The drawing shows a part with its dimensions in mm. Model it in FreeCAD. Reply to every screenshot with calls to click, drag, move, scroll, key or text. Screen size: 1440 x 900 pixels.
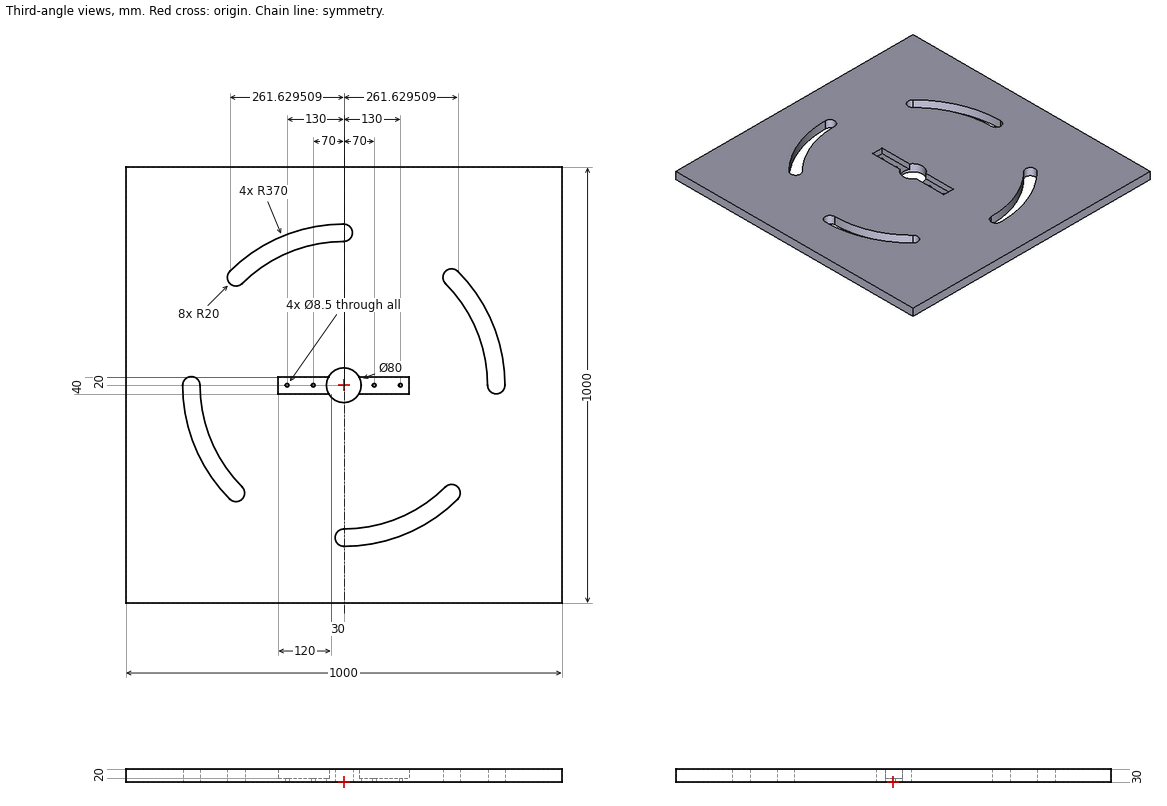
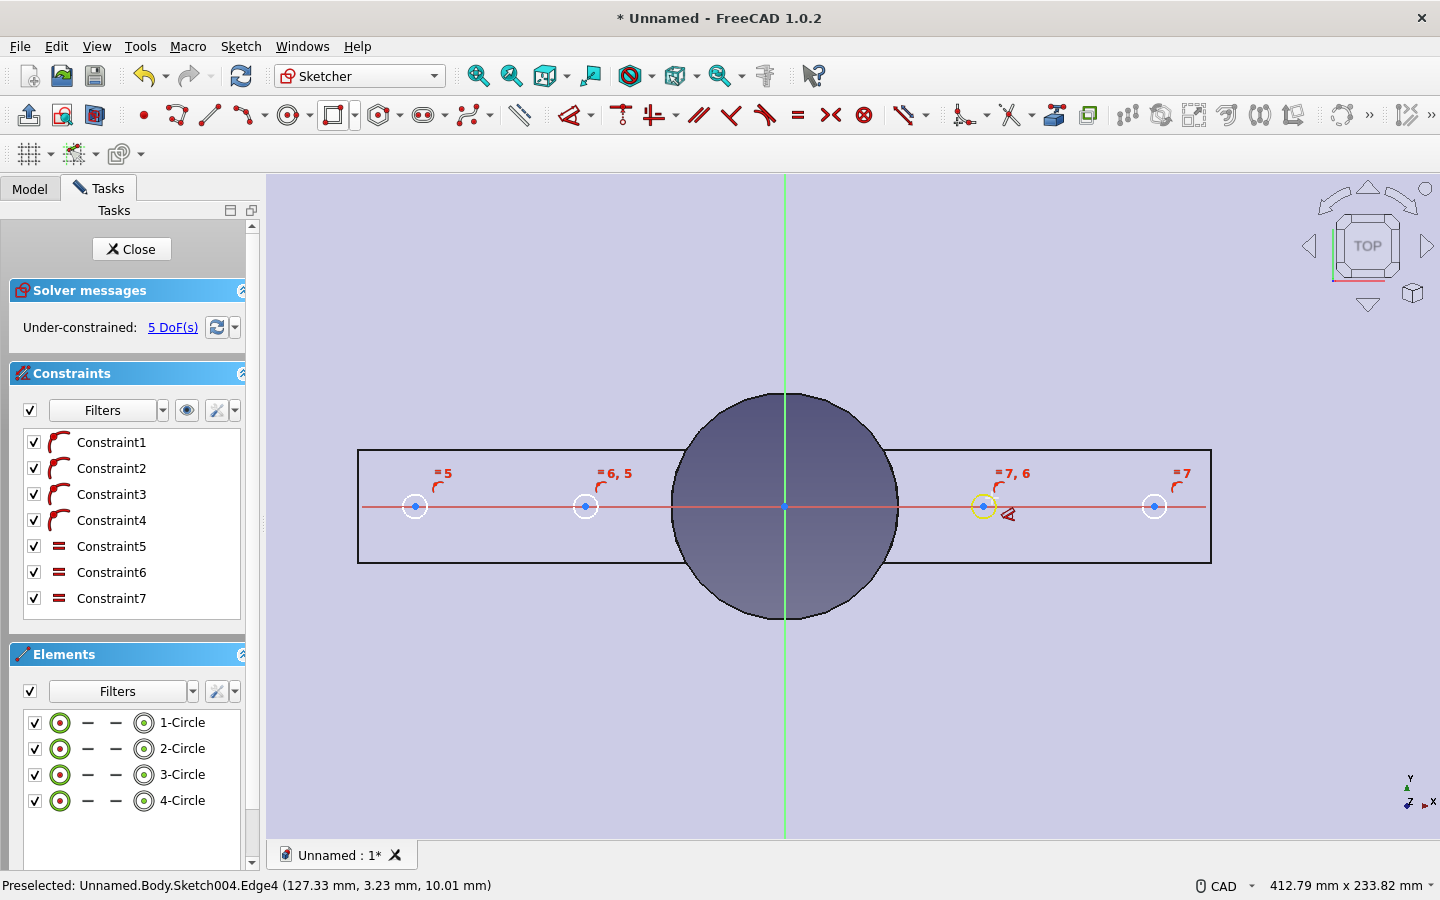
scroll(423, 498, up, 3)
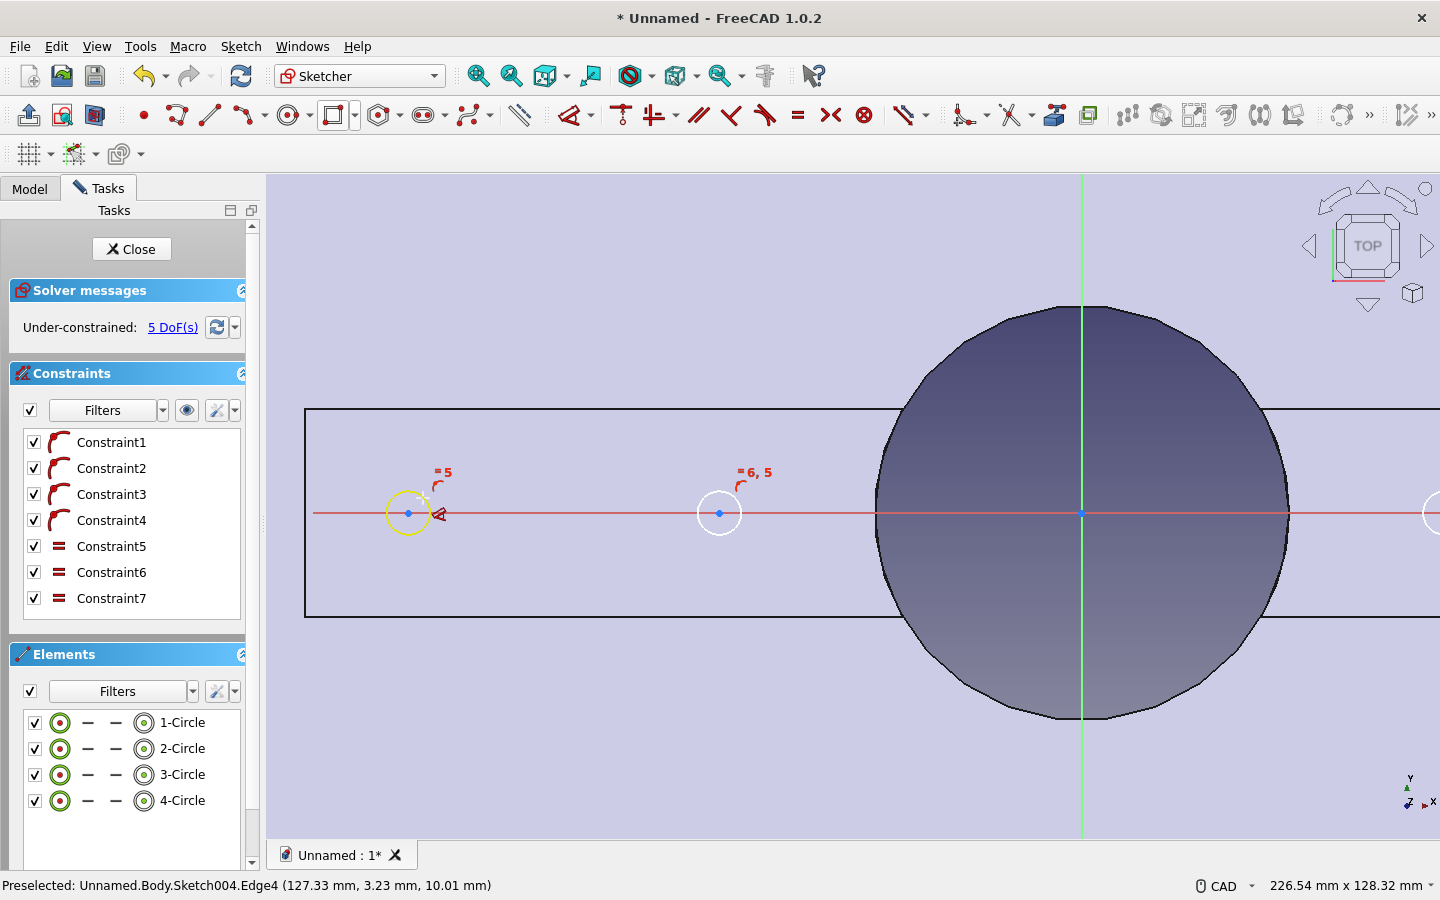
click(424, 498)
click(447, 476)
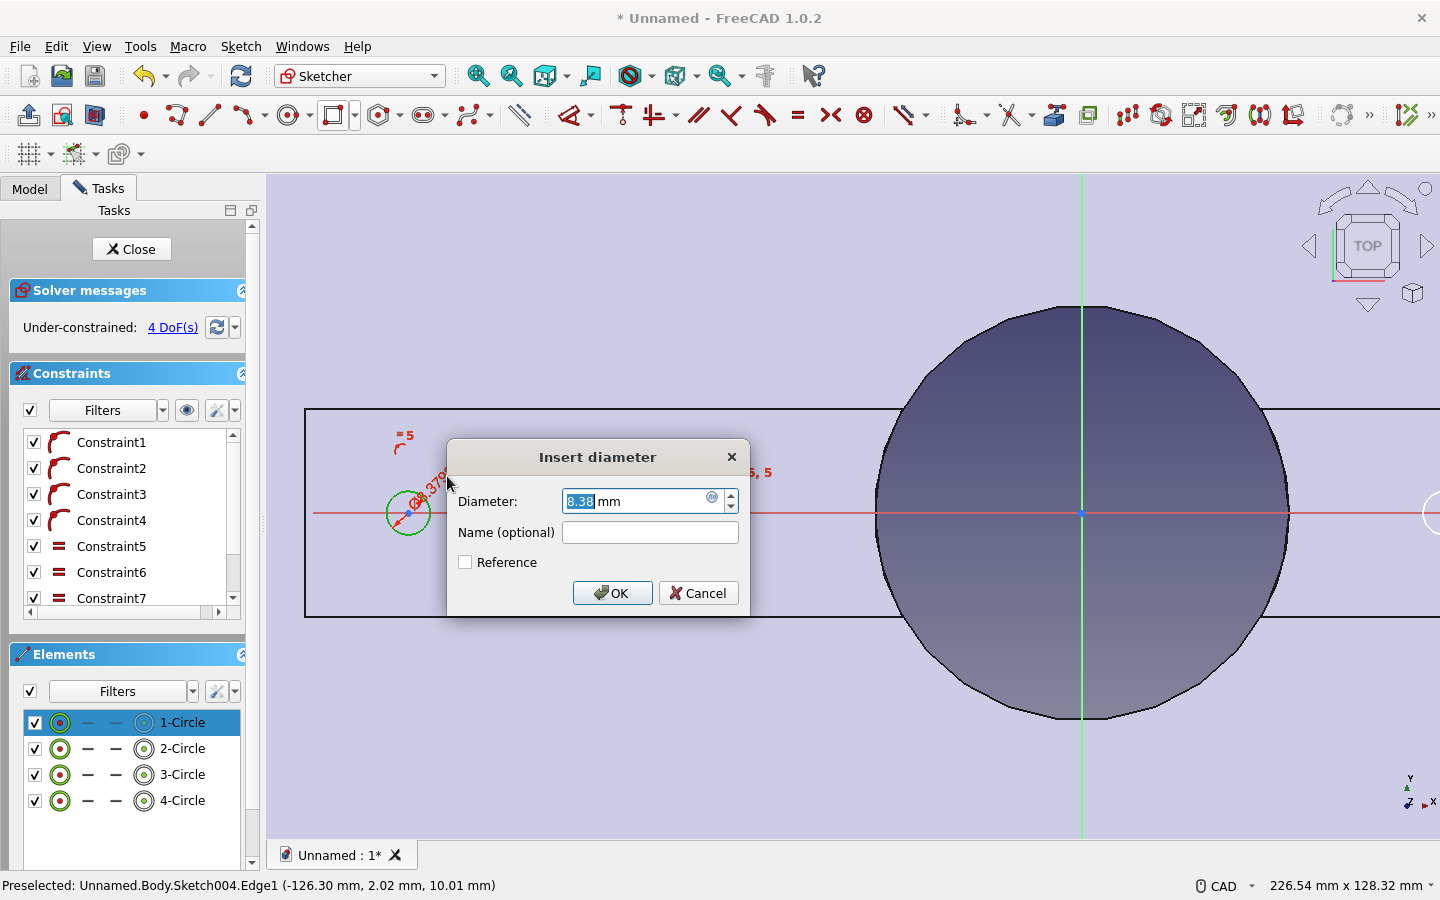
text(8.5)
key(Return)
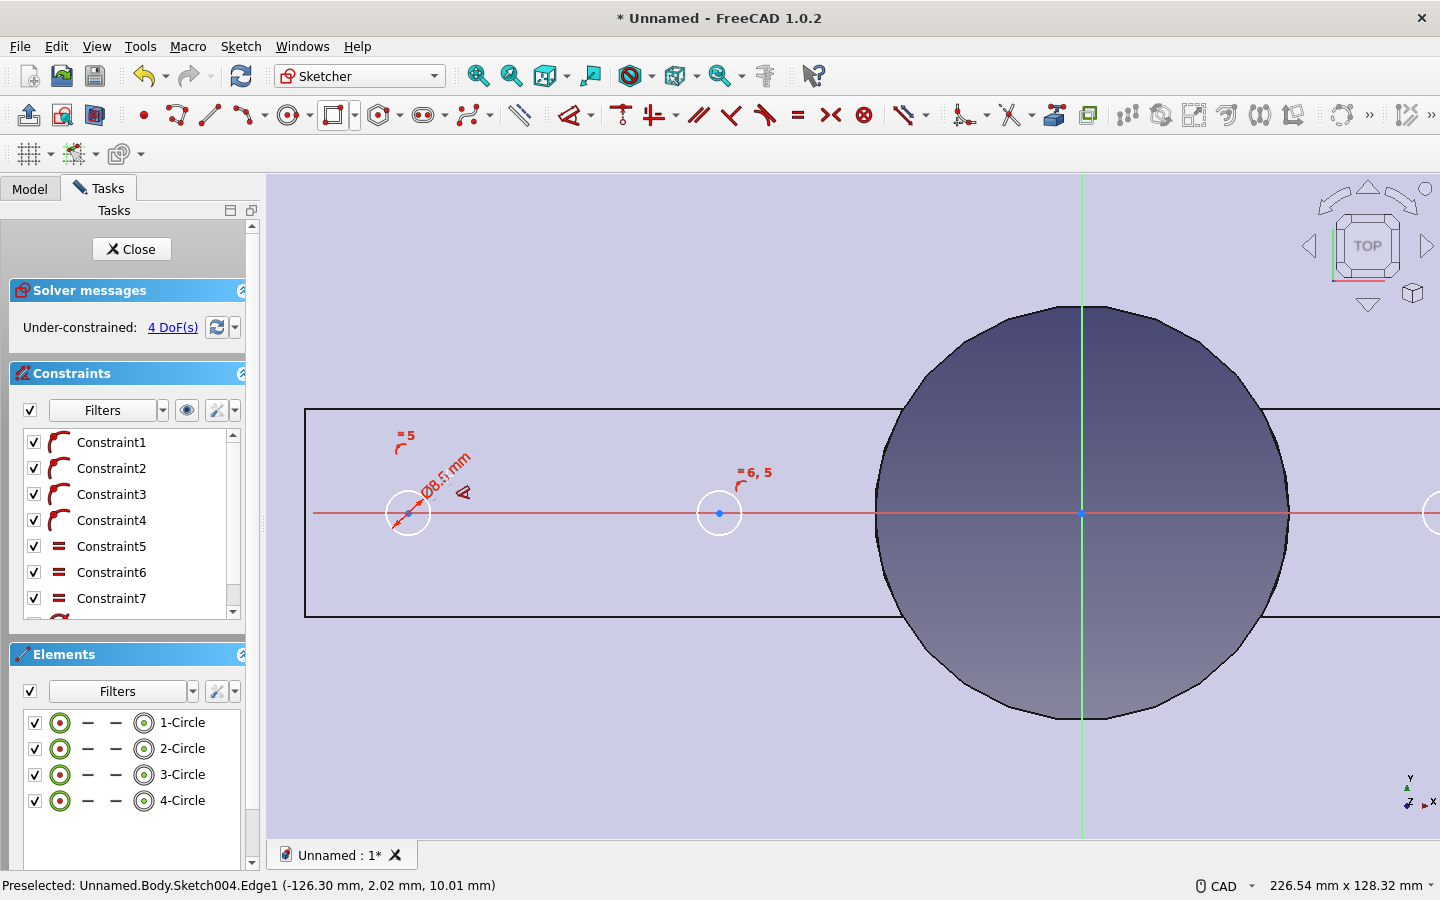
click(719, 513)
click(901, 547)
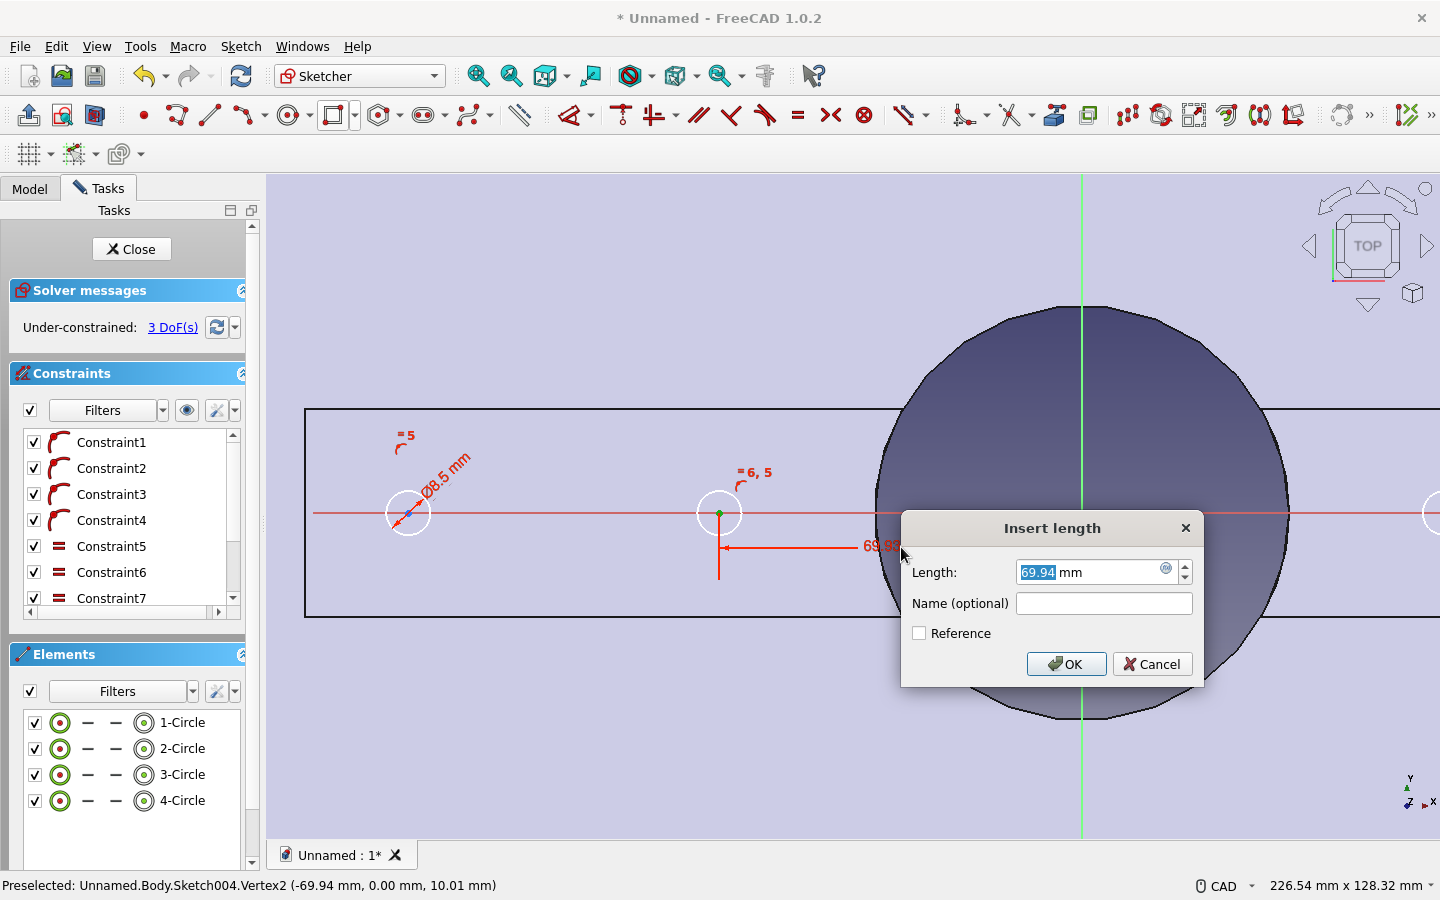
text(70)
key(Return)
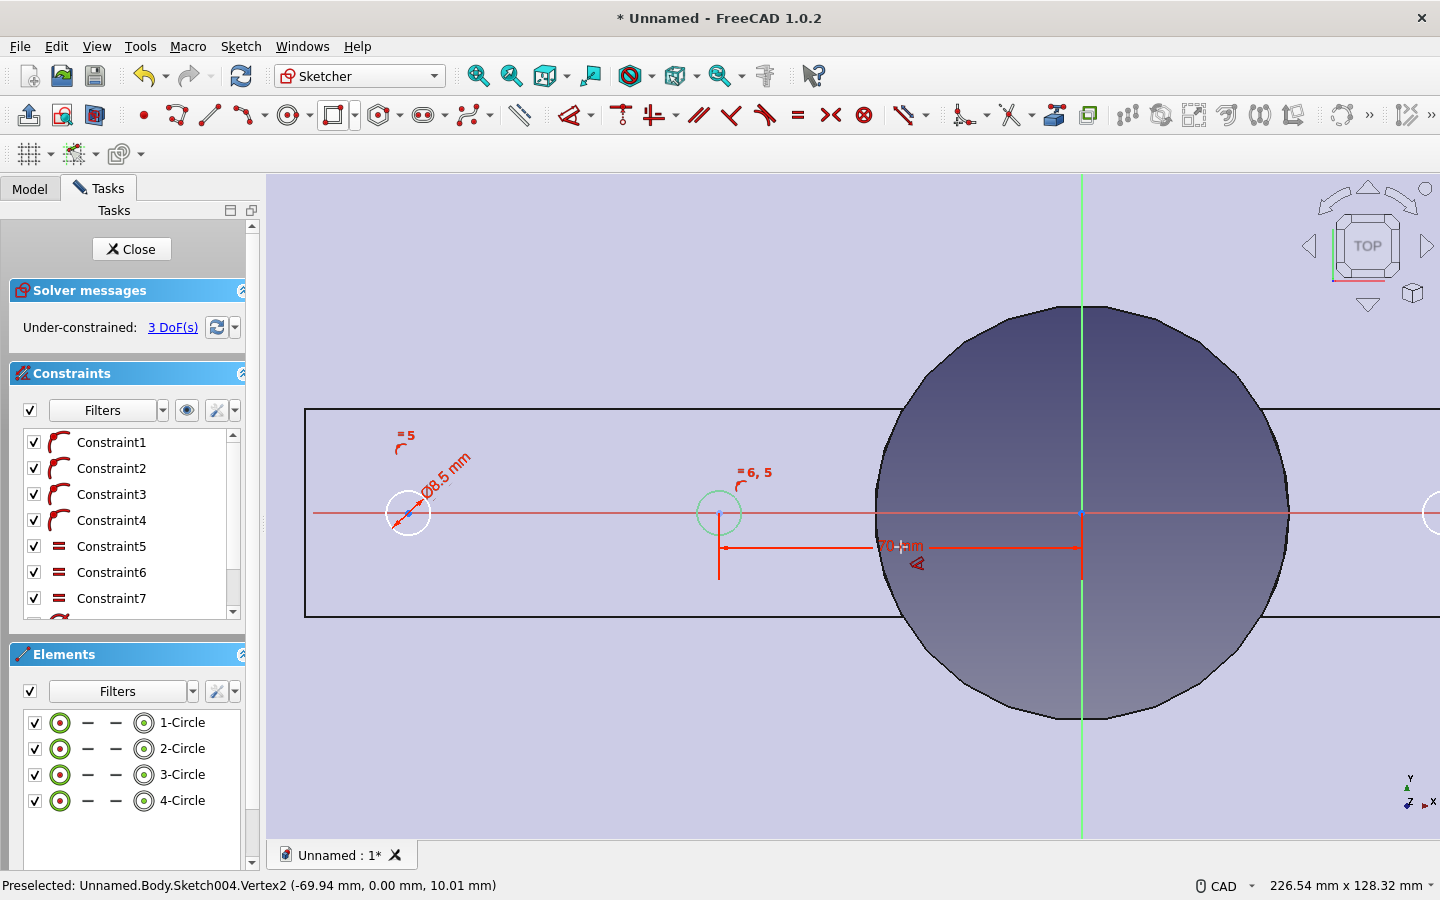
scroll(423, 498, down, 3)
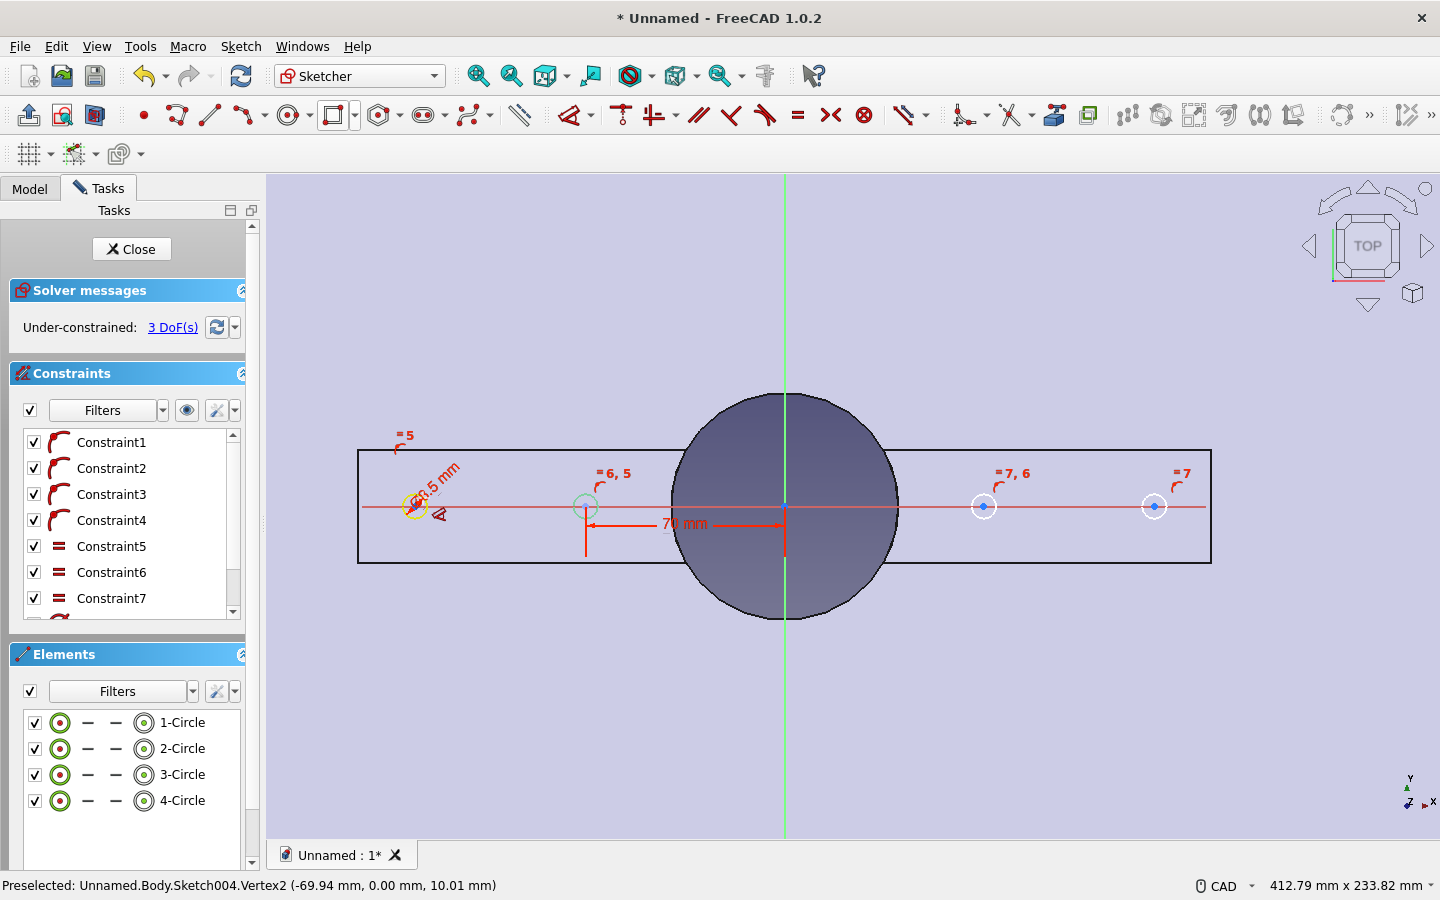
click(984, 506)
click(884, 540)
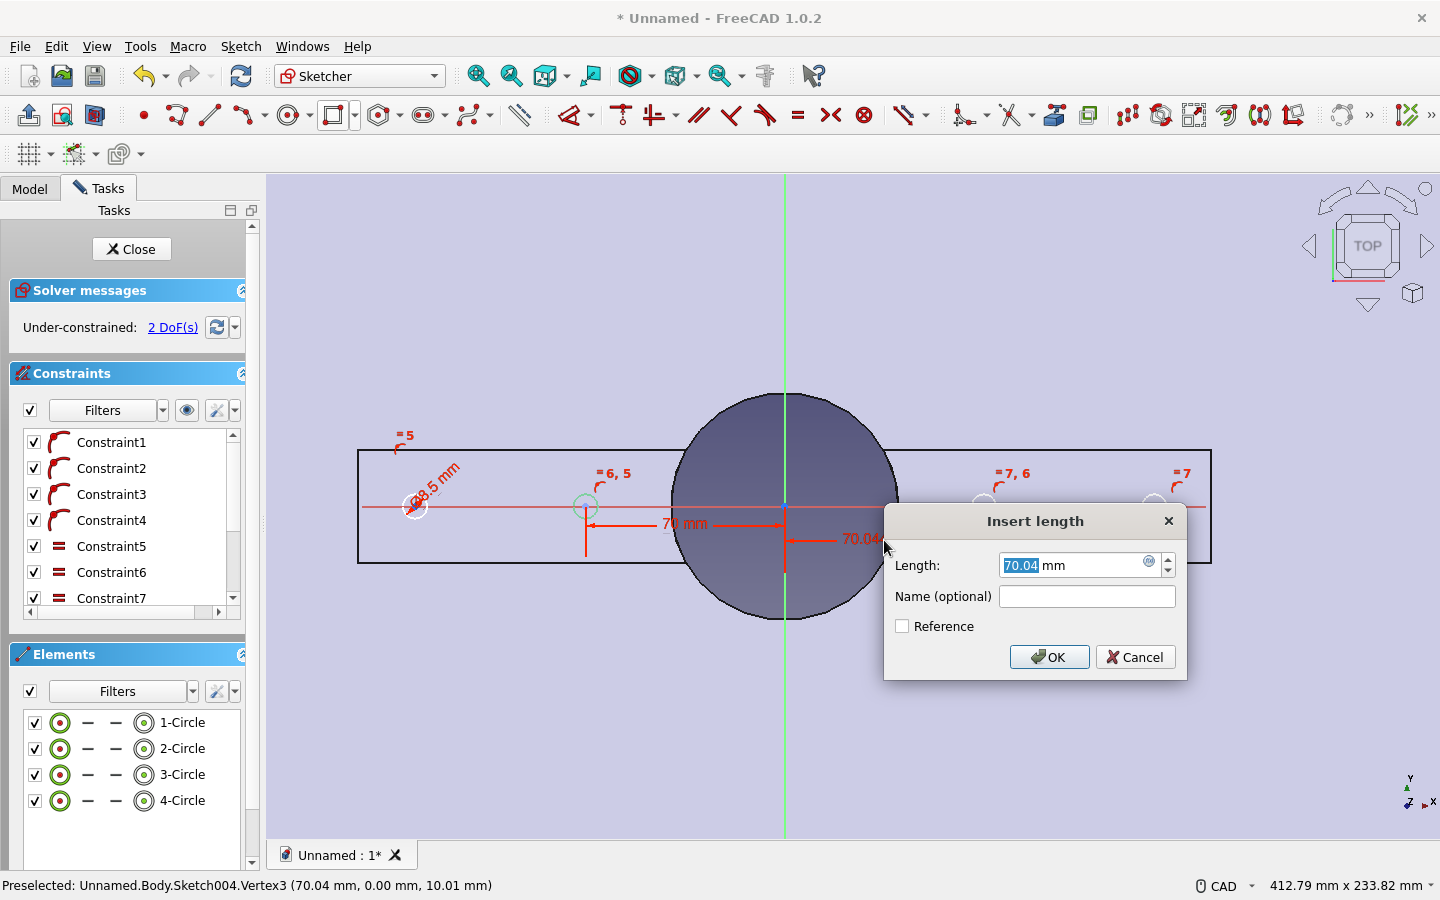
text(70)
key(Return)